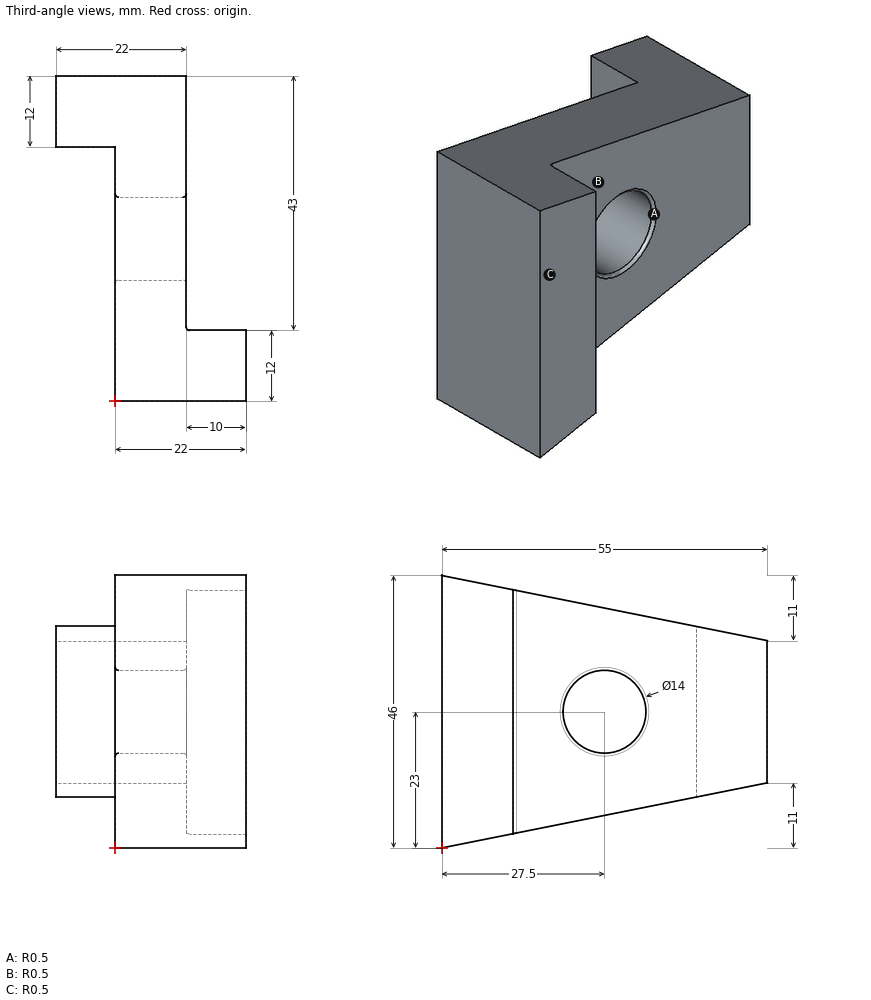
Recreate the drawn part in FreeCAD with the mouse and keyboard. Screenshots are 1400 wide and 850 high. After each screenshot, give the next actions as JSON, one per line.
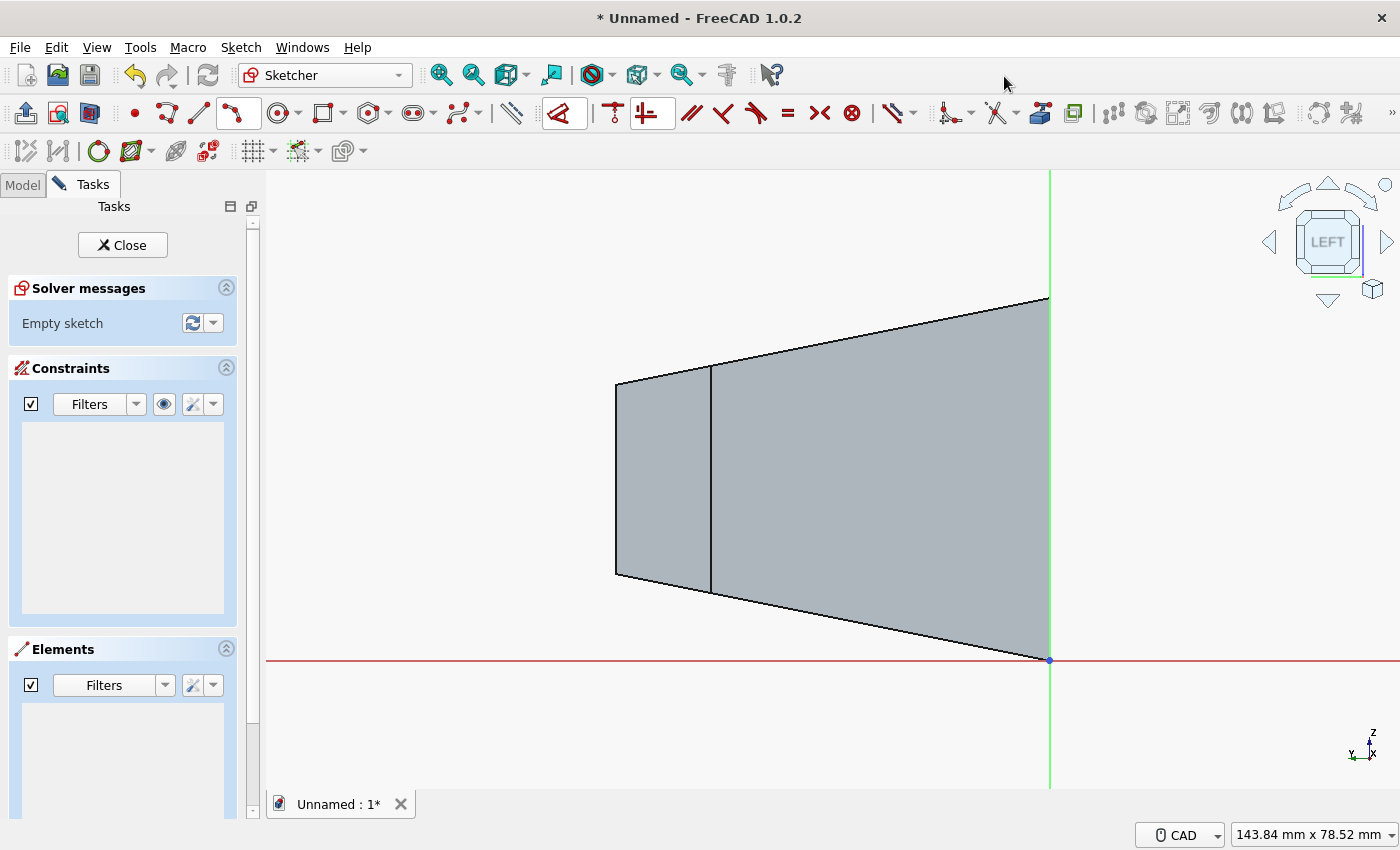
{"action": "scroll", "coordinate": [1095, 619], "scroll_direction": "up", "scroll_amount": 3}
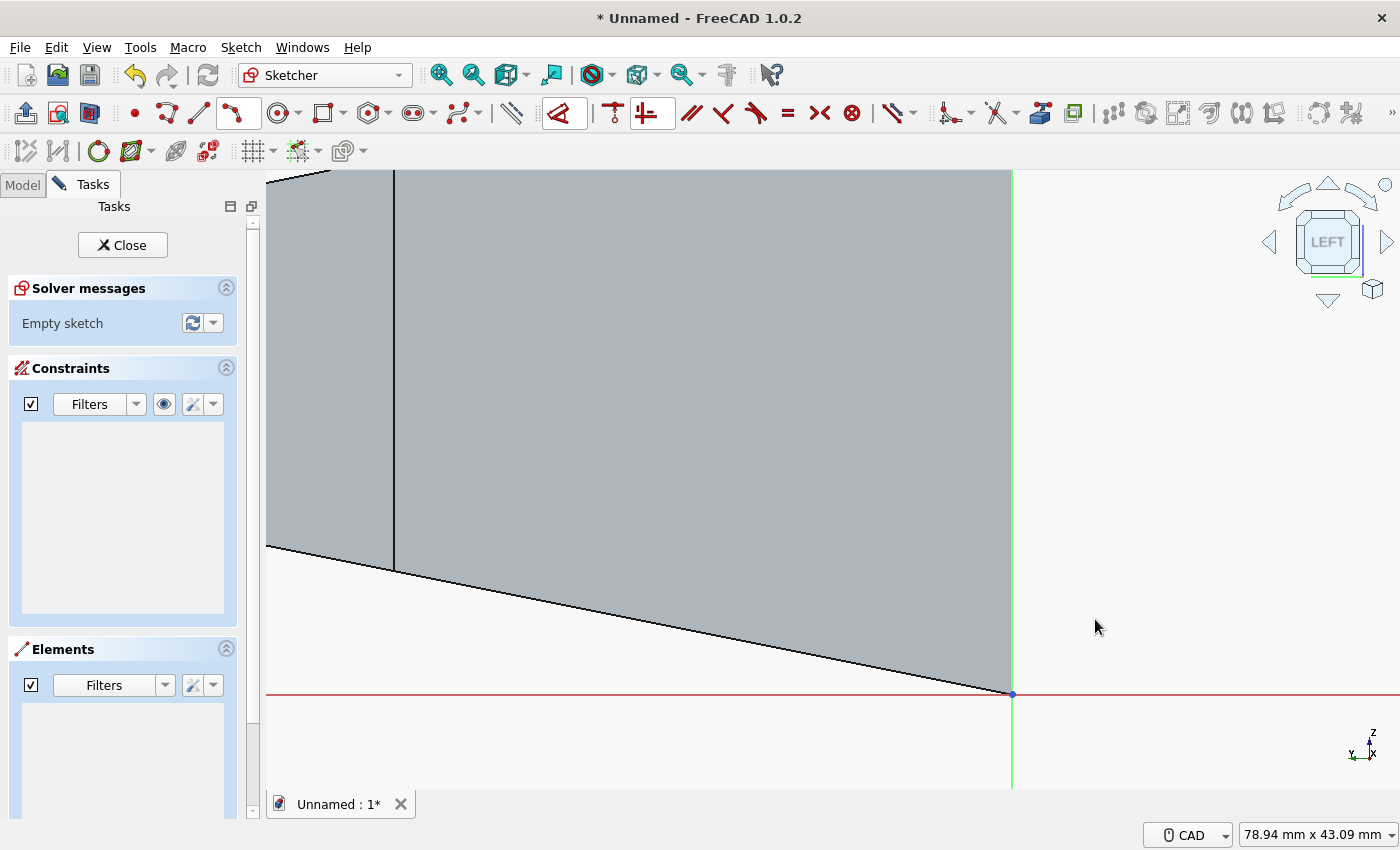
{"action": "left_click", "coordinate": [278, 114]}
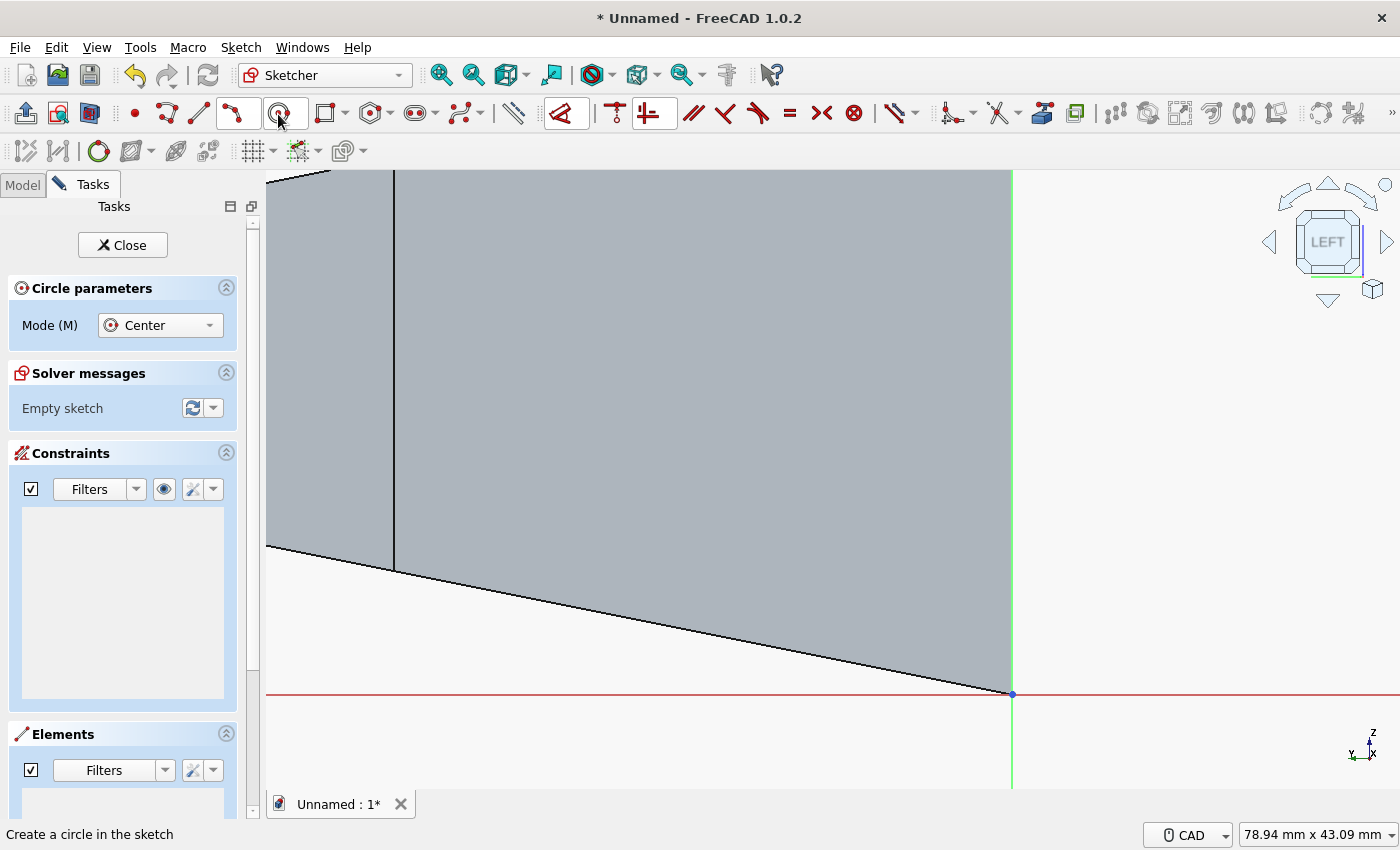
{"action": "left_click", "coordinate": [617, 364]}
{"action": "mouse_move", "coordinate": [688, 293]}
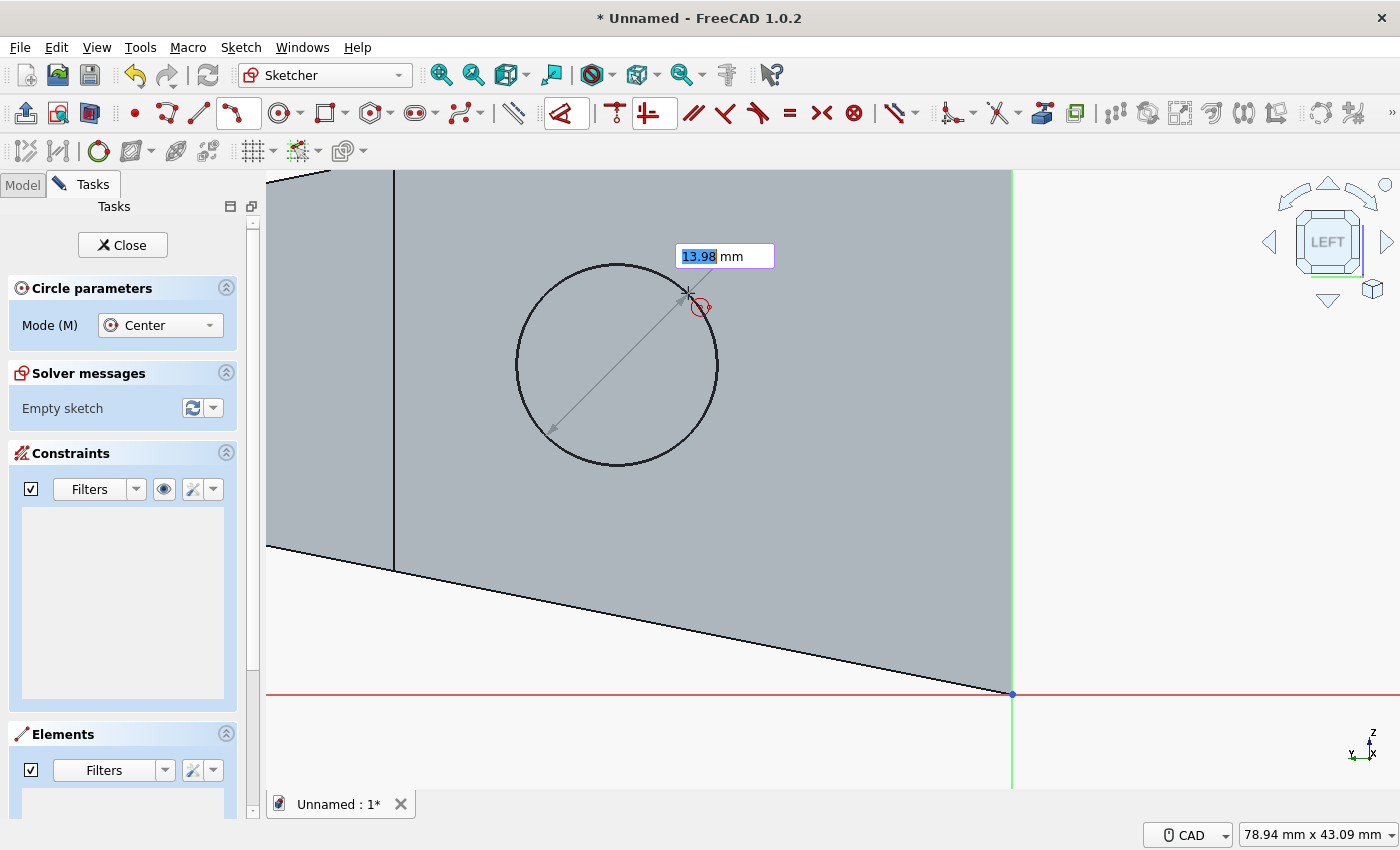
{"action": "type", "text": "14"}
{"action": "key", "text": "Return"}
{"action": "key", "text": "Escape"}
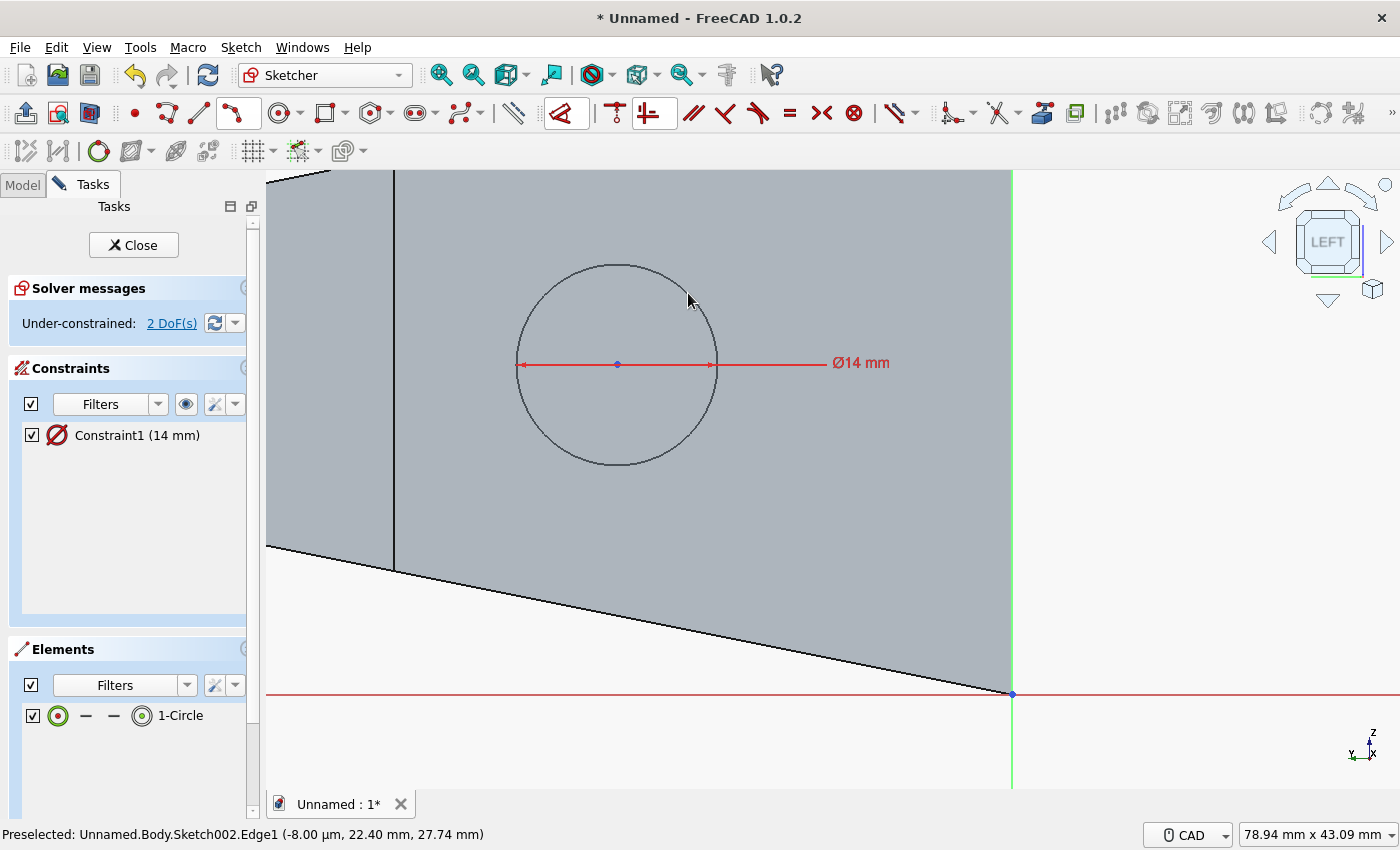
{"action": "left_click", "coordinate": [617, 365]}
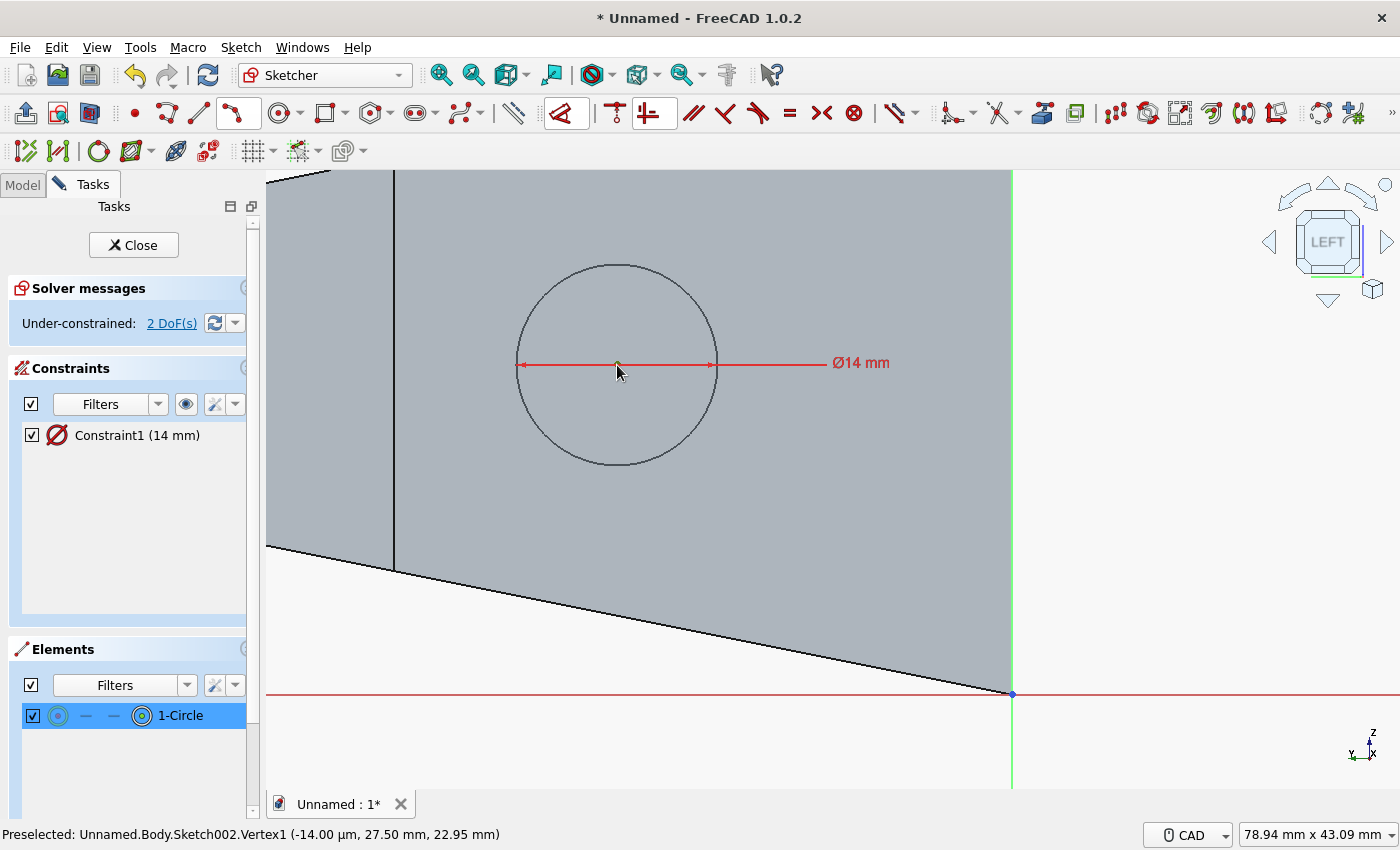
{"action": "left_click", "coordinate": [584, 114]}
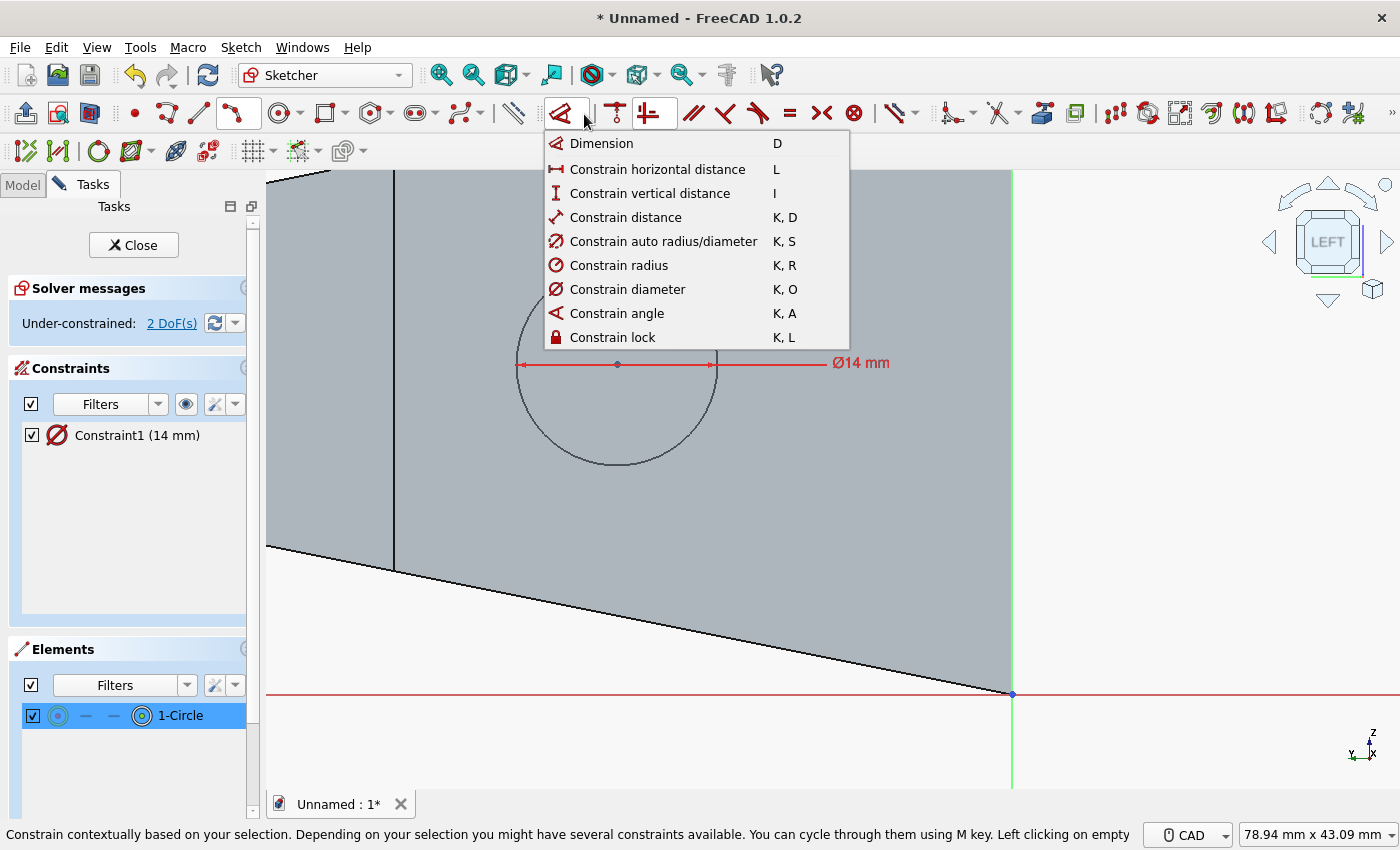
{"action": "left_click", "coordinate": [697, 193]}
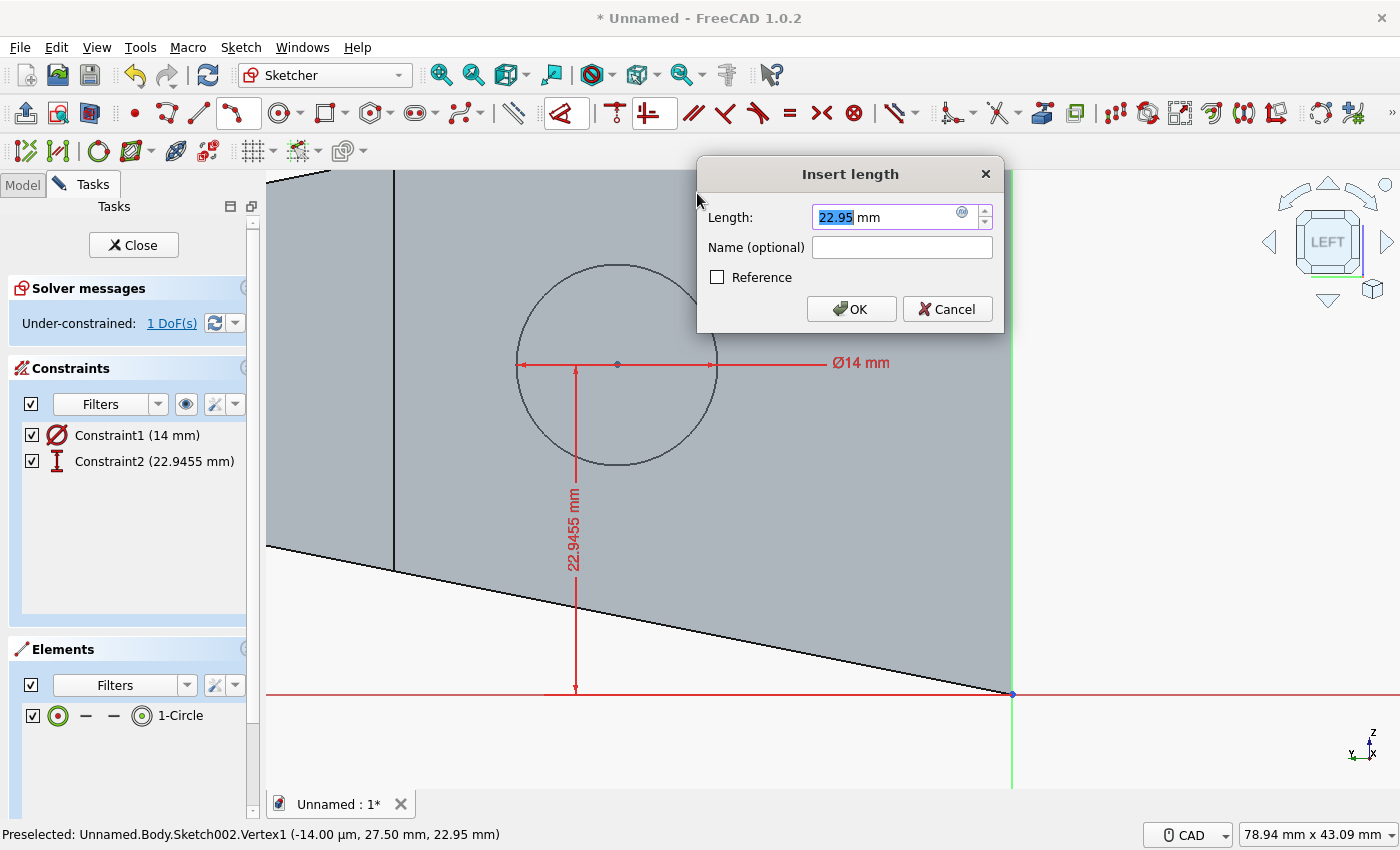
{"action": "type", "text": "23"}
{"action": "key", "text": "Return"}